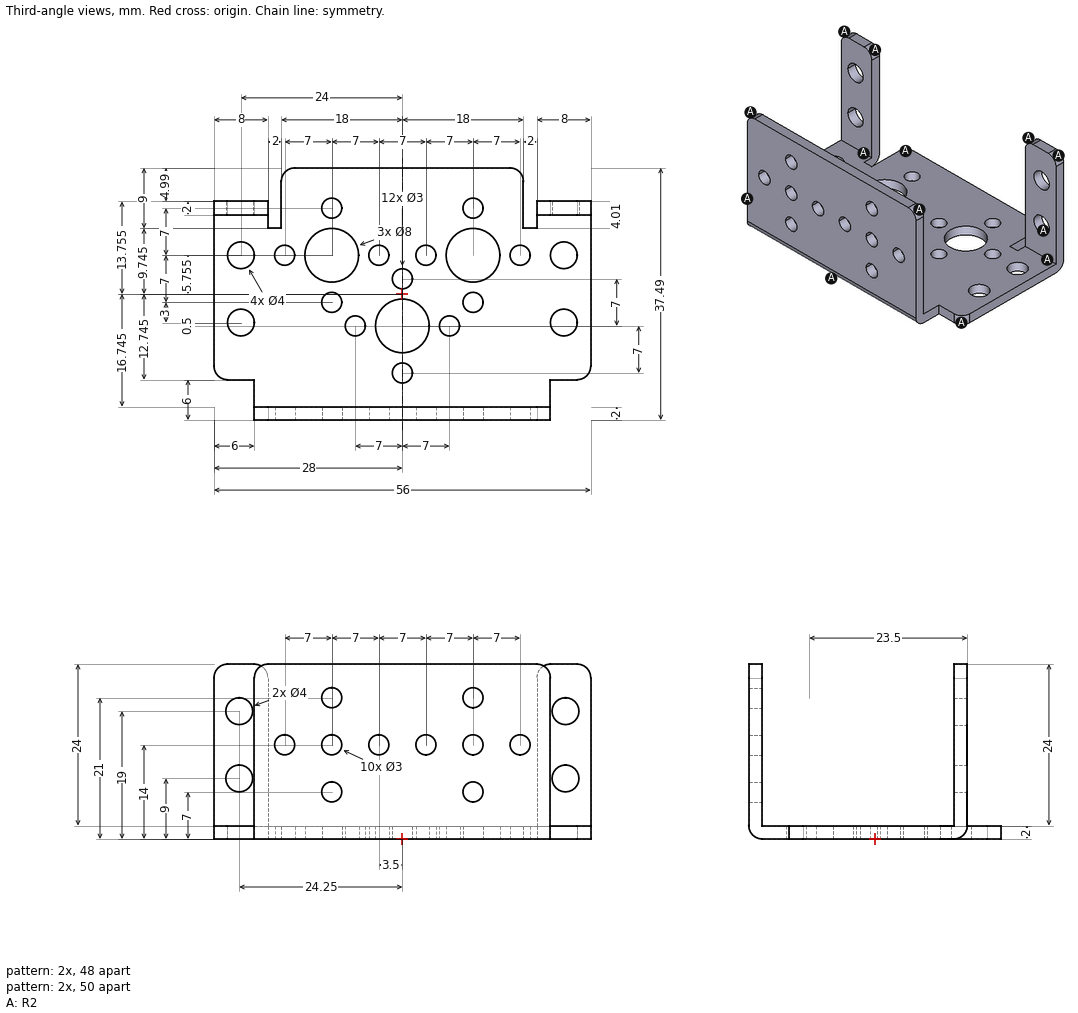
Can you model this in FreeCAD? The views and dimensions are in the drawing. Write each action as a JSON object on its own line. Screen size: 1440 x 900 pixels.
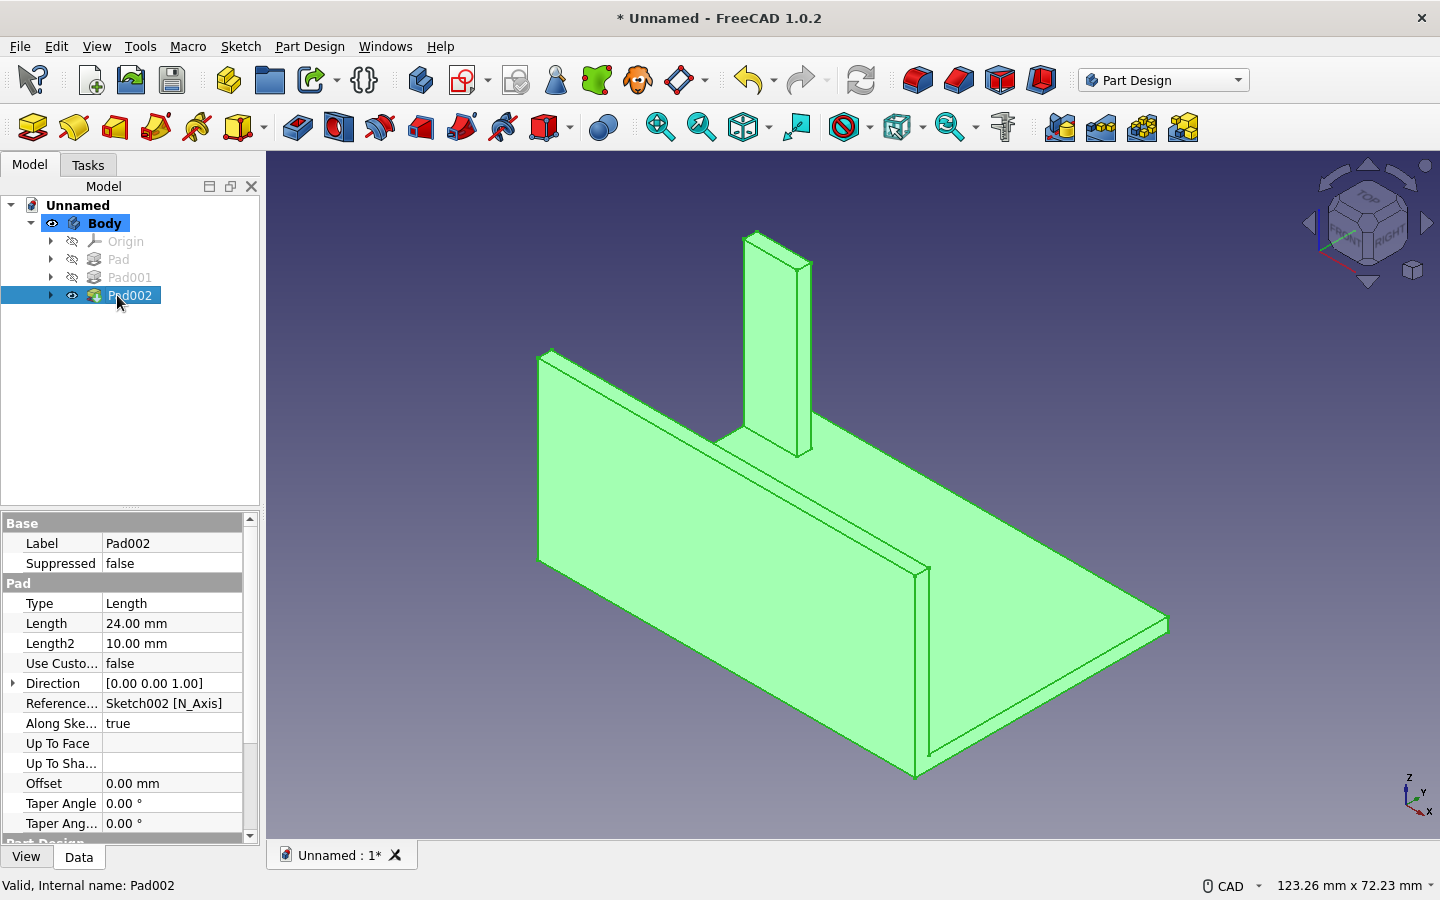
{"action": "left_click", "coordinate": [1101, 128]}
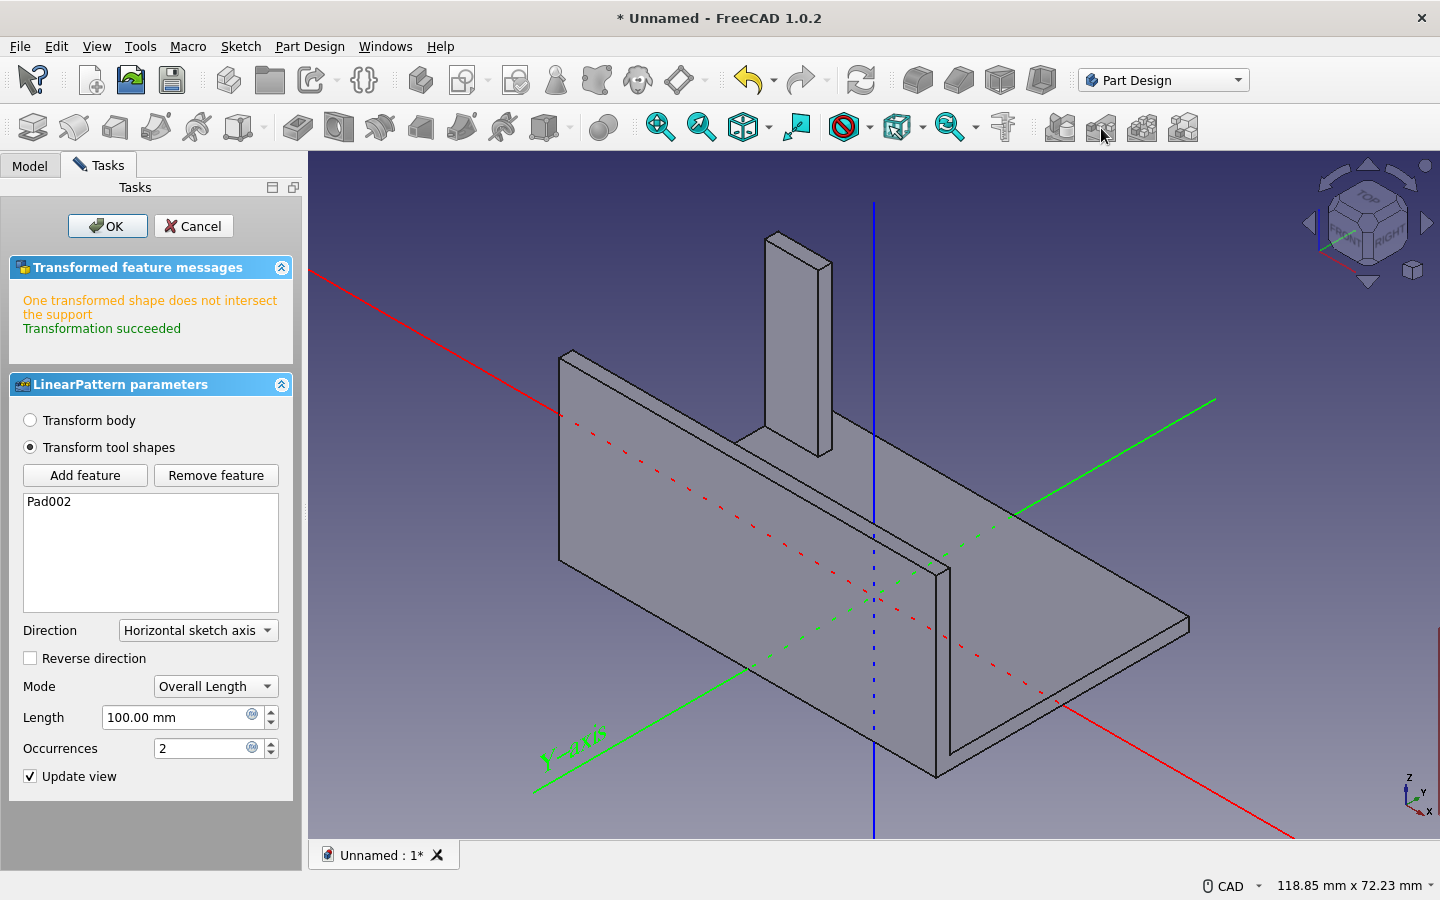
{"action": "left_click", "coordinate": [199, 630]}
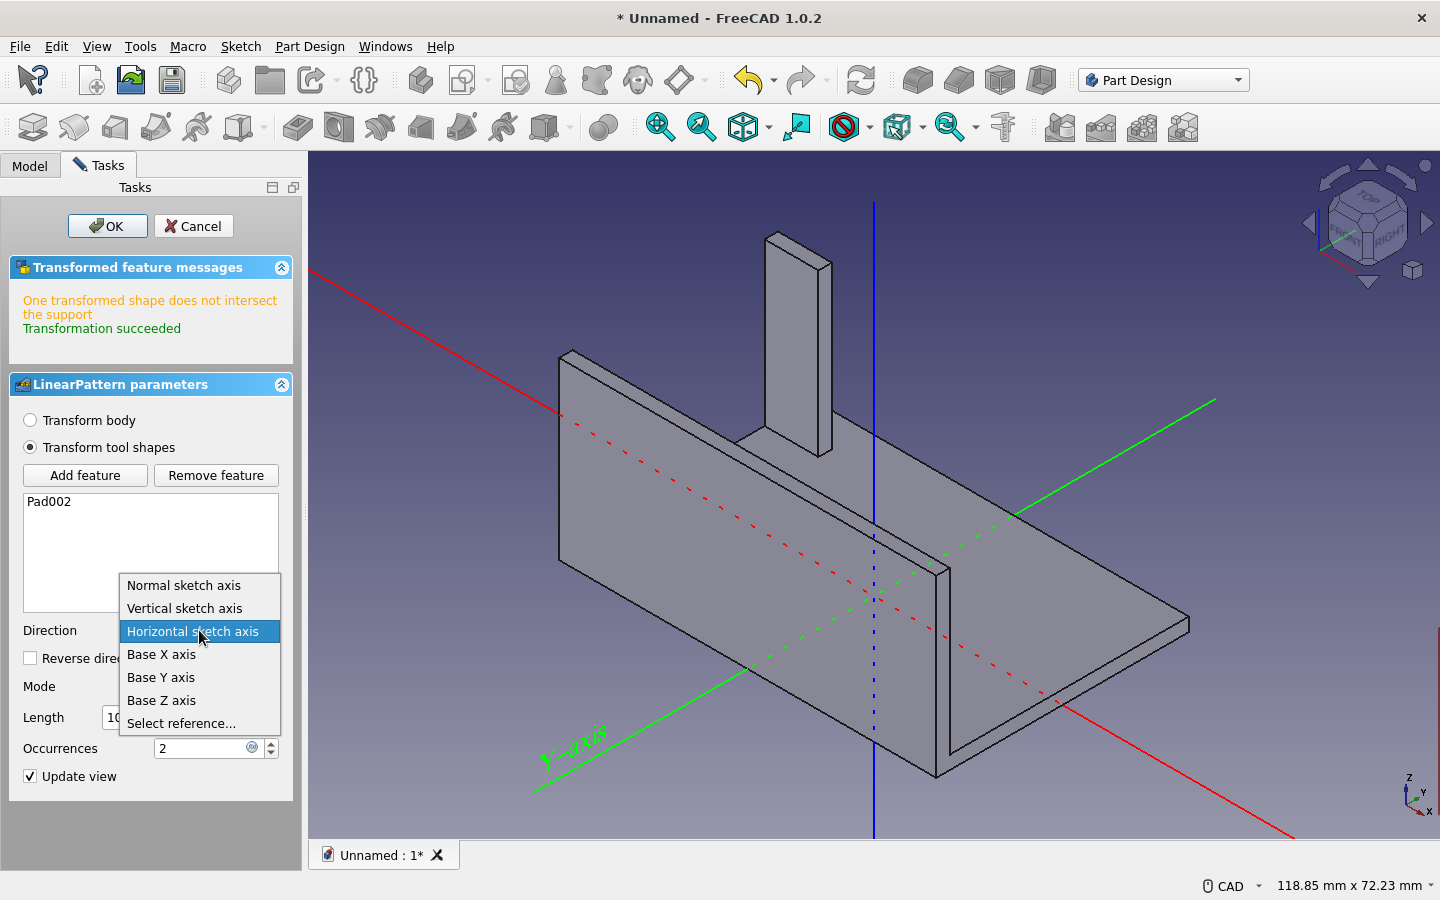
{"action": "left_click", "coordinate": [198, 654]}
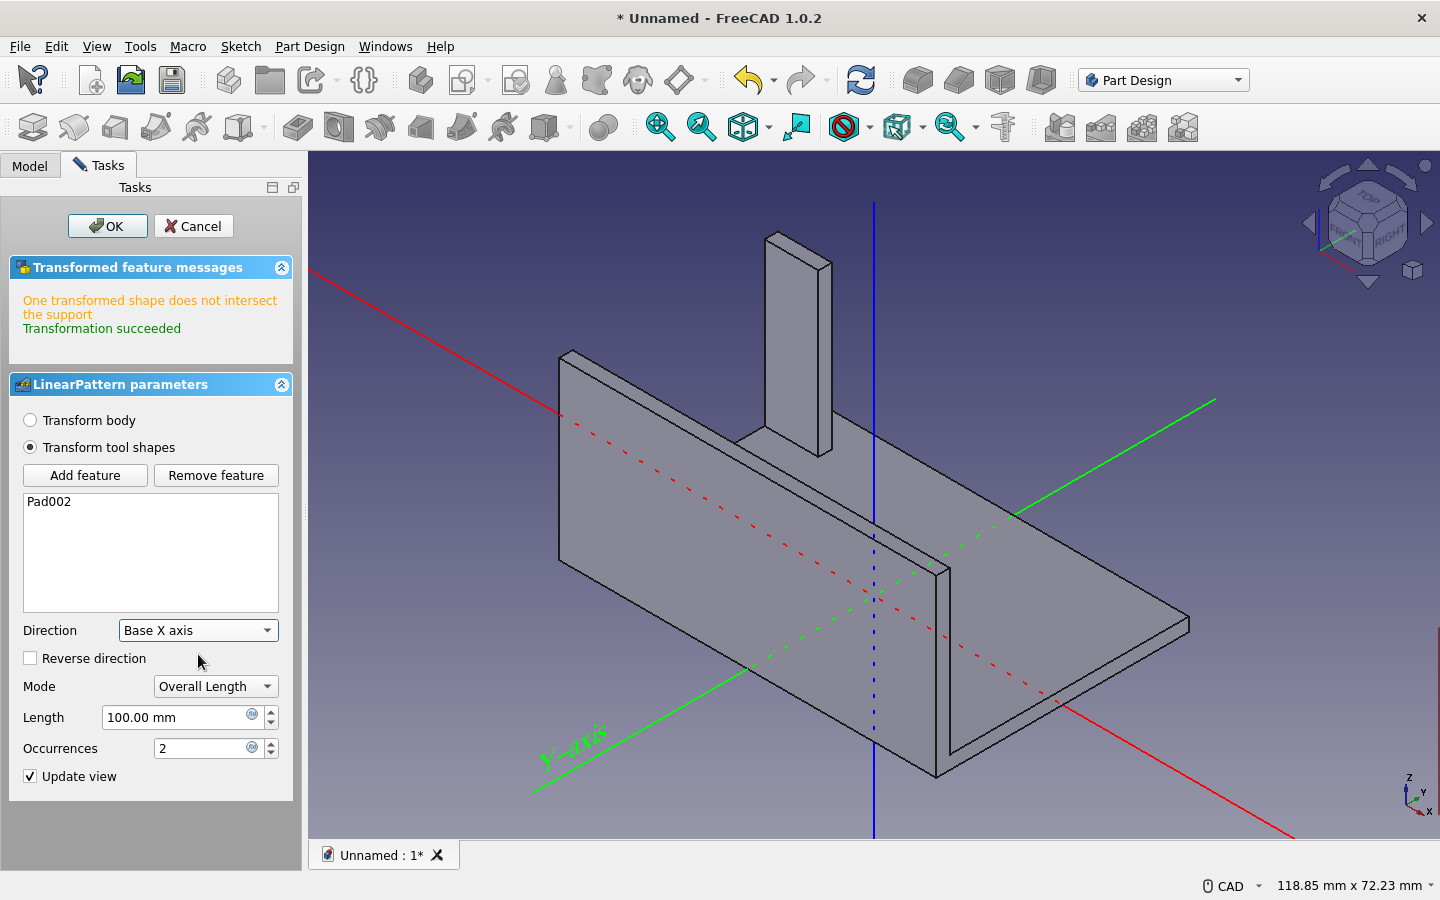
{"action": "left_click", "coordinate": [216, 686]}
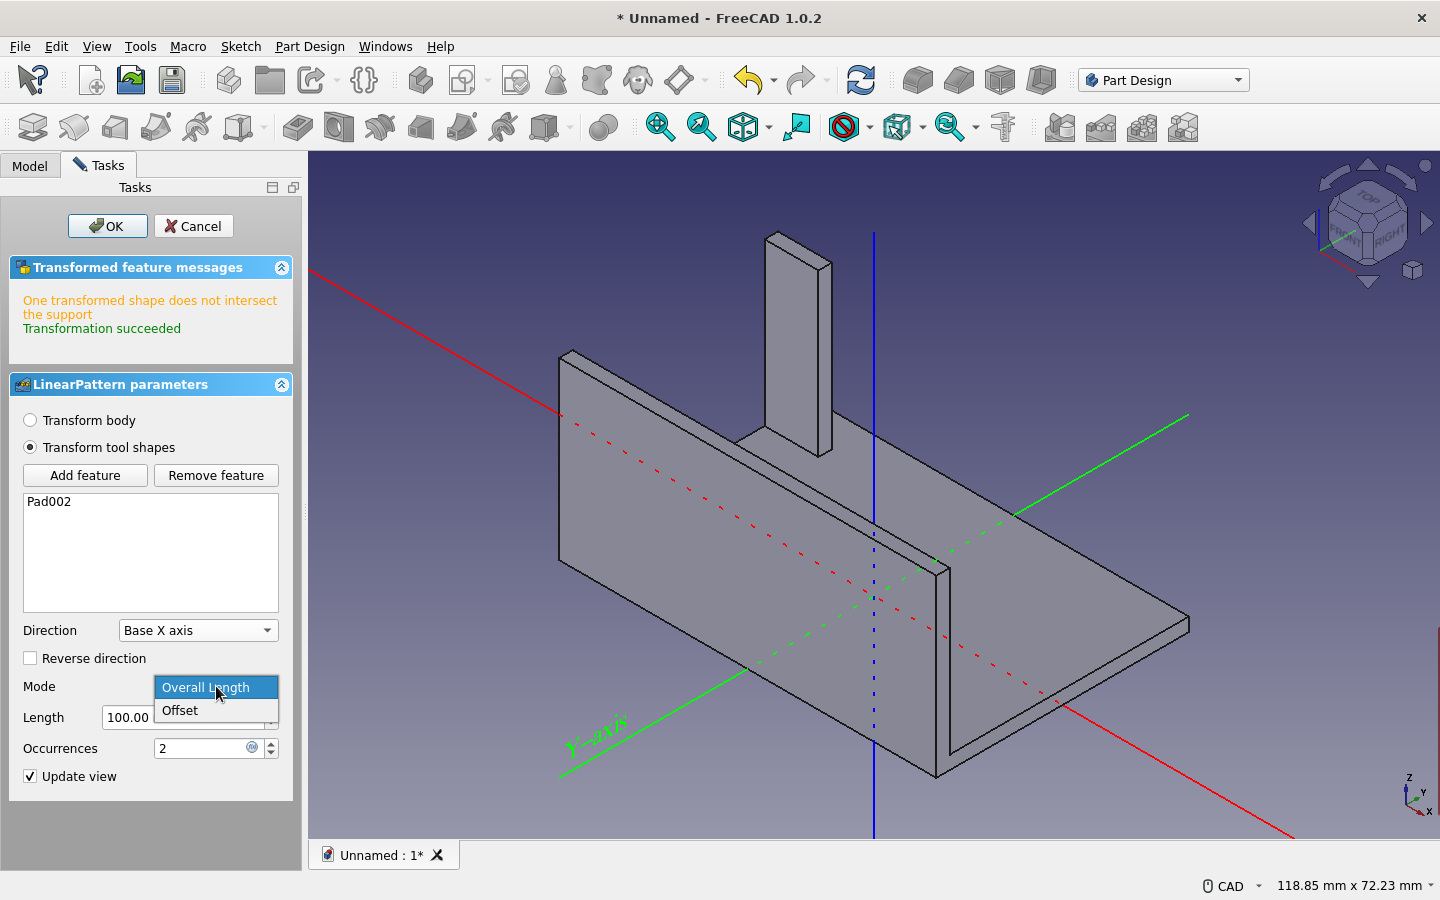
{"action": "left_click", "coordinate": [214, 710]}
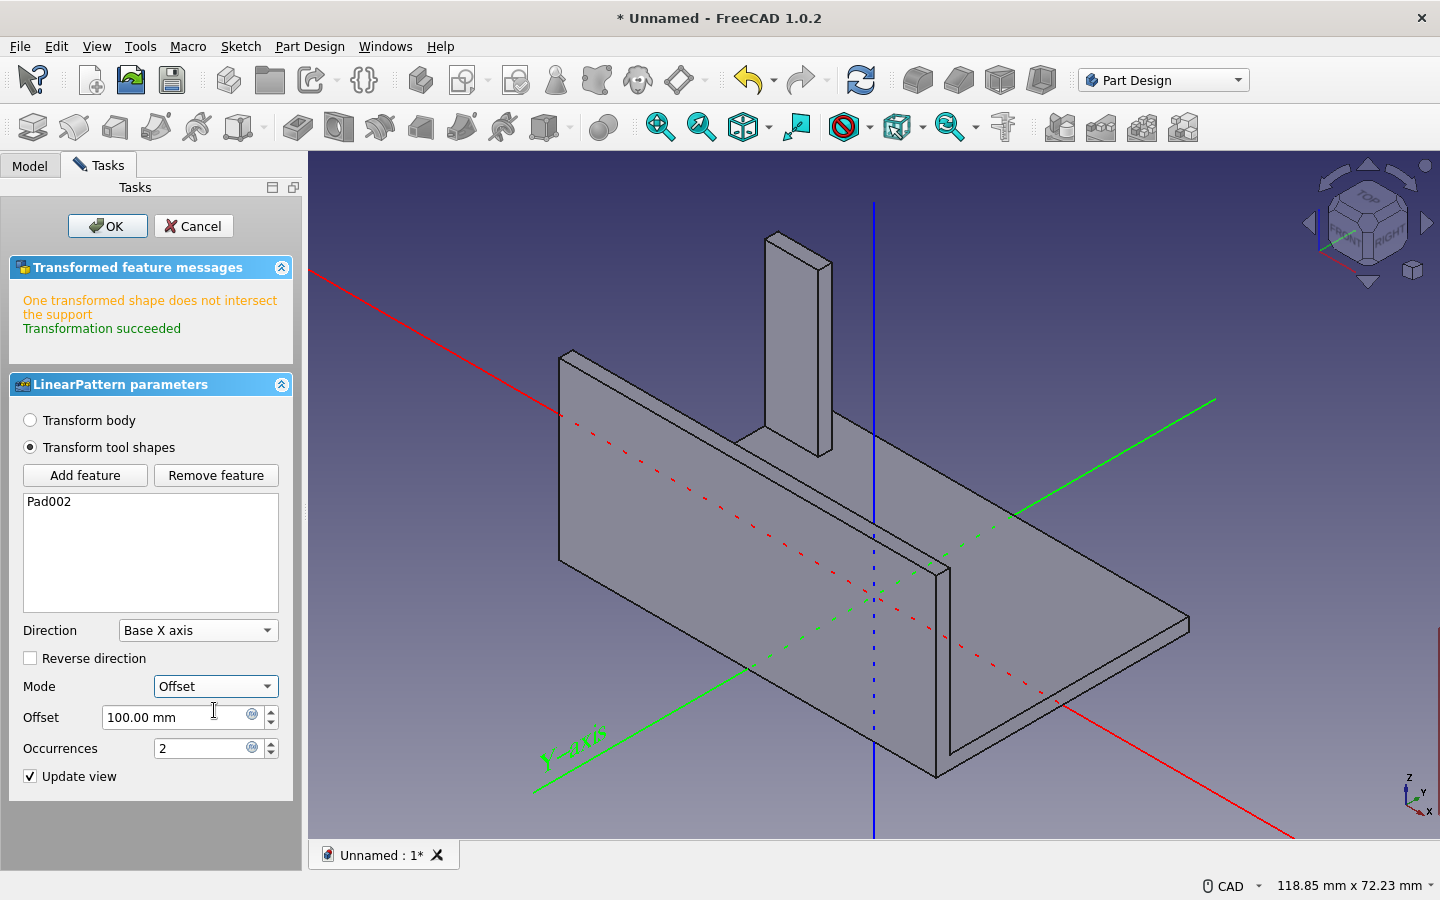
{"action": "triple_click", "coordinate": [184, 718]}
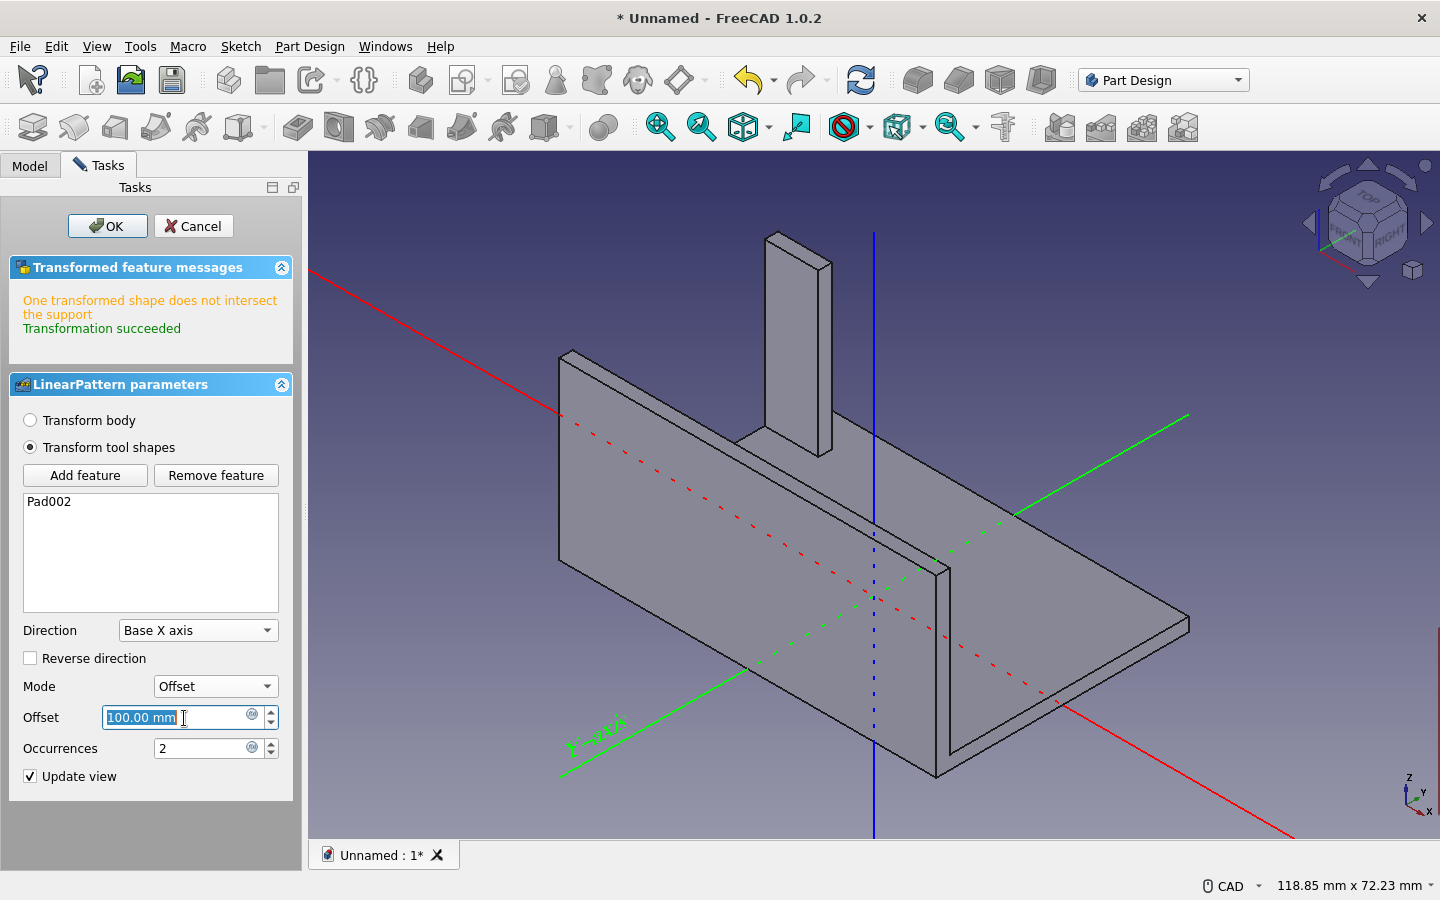
{"action": "type", "text": "48"}
{"action": "key", "text": "Tab"}